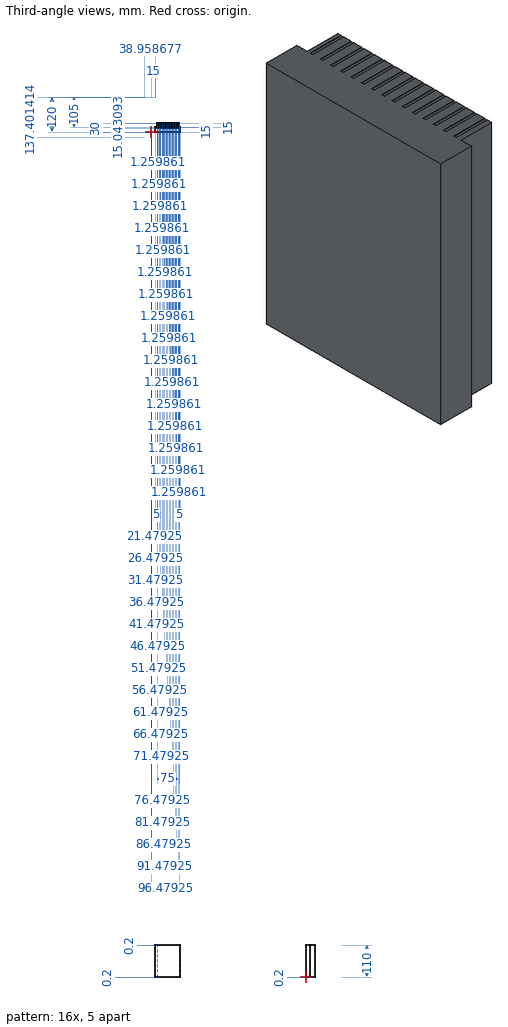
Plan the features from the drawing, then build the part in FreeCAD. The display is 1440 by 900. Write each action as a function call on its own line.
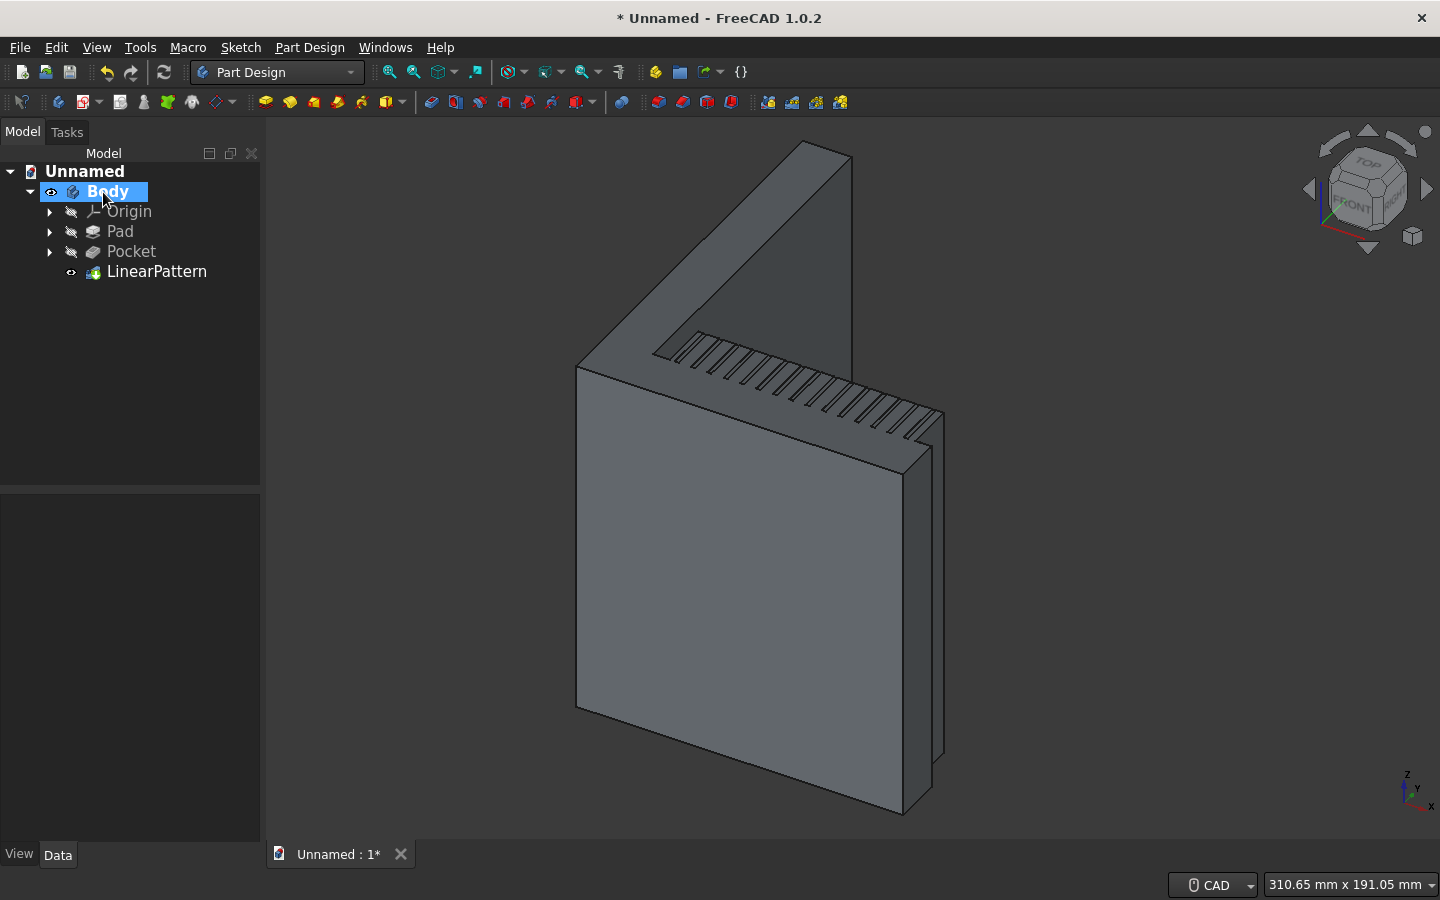
click(50, 212)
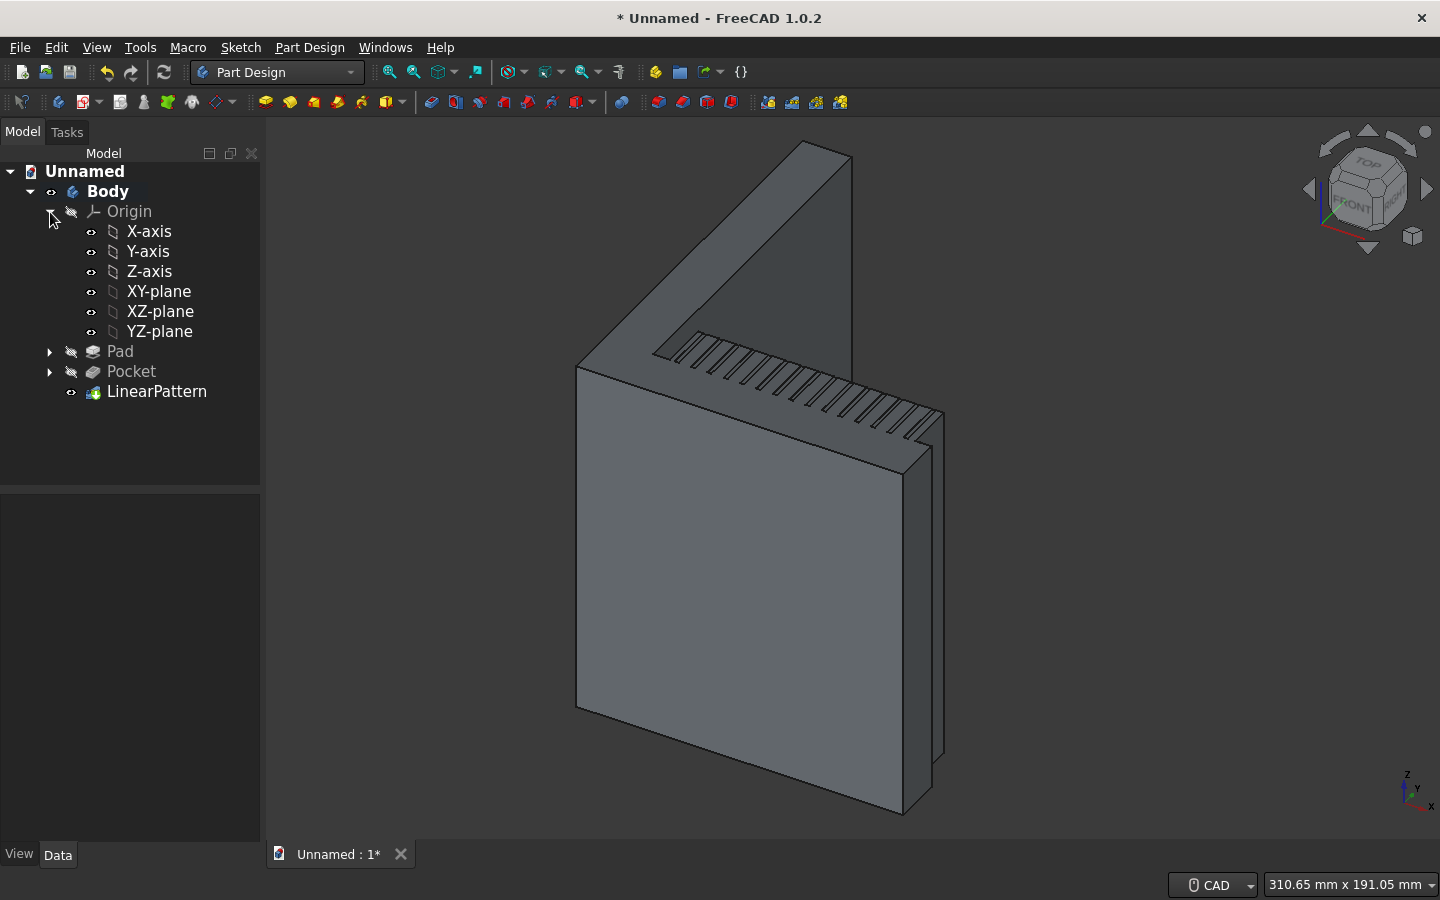
click(136, 292)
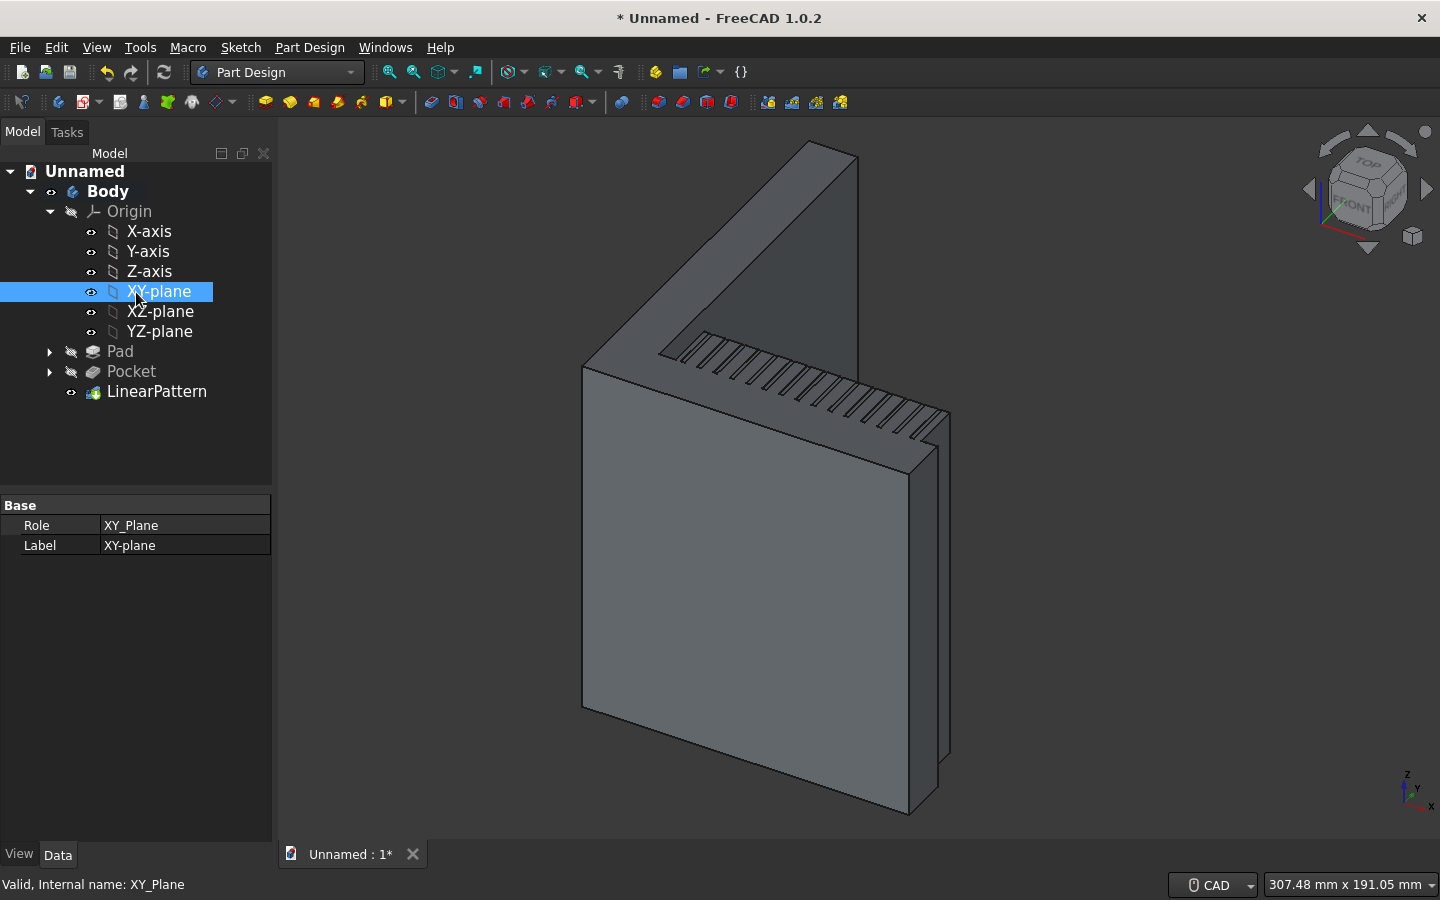
click(216, 102)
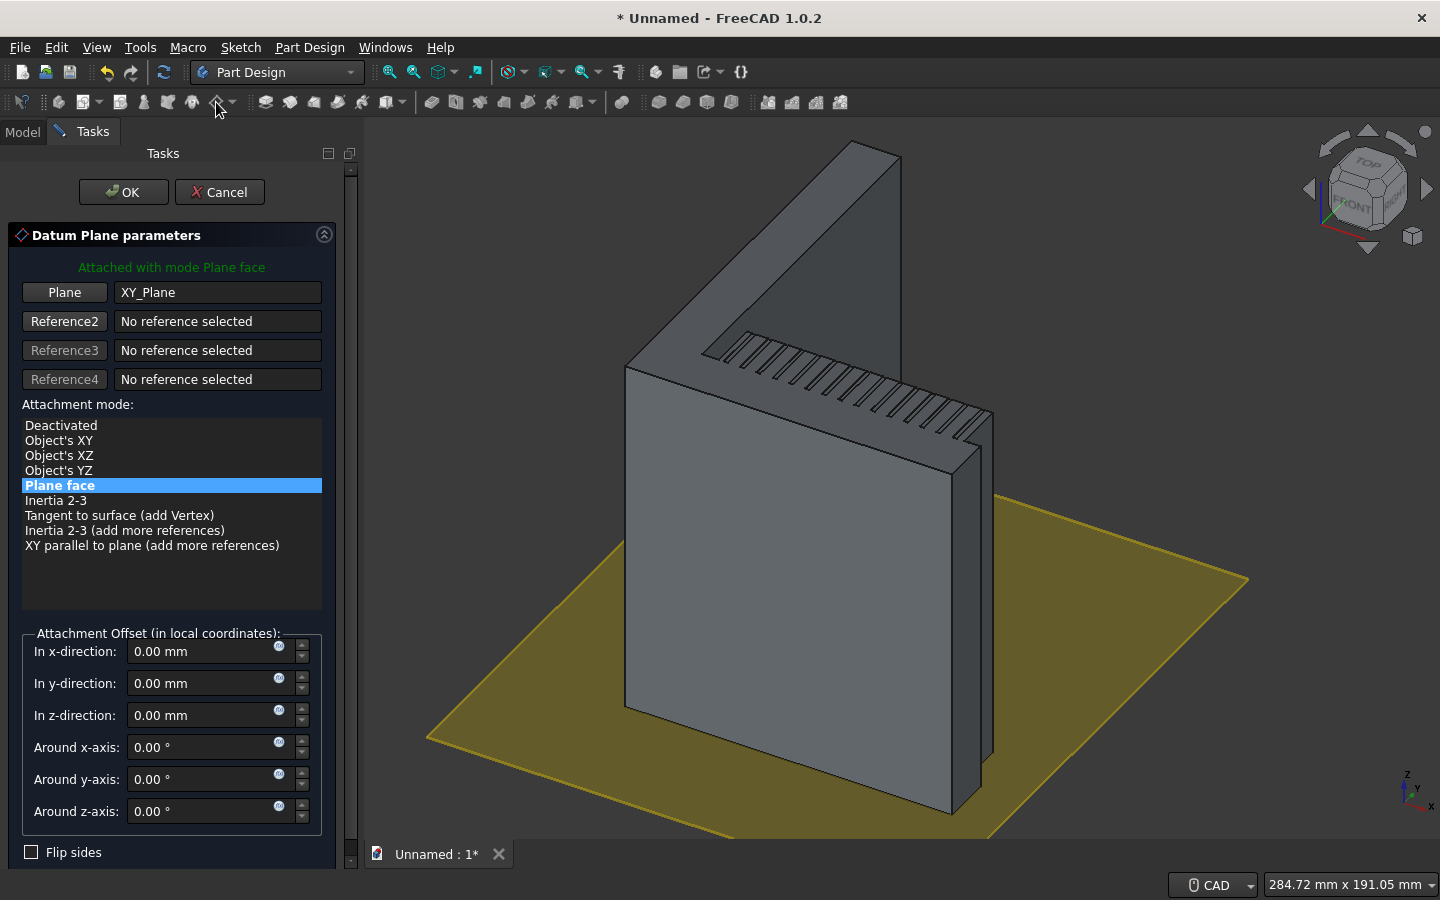
triple_click(210, 715)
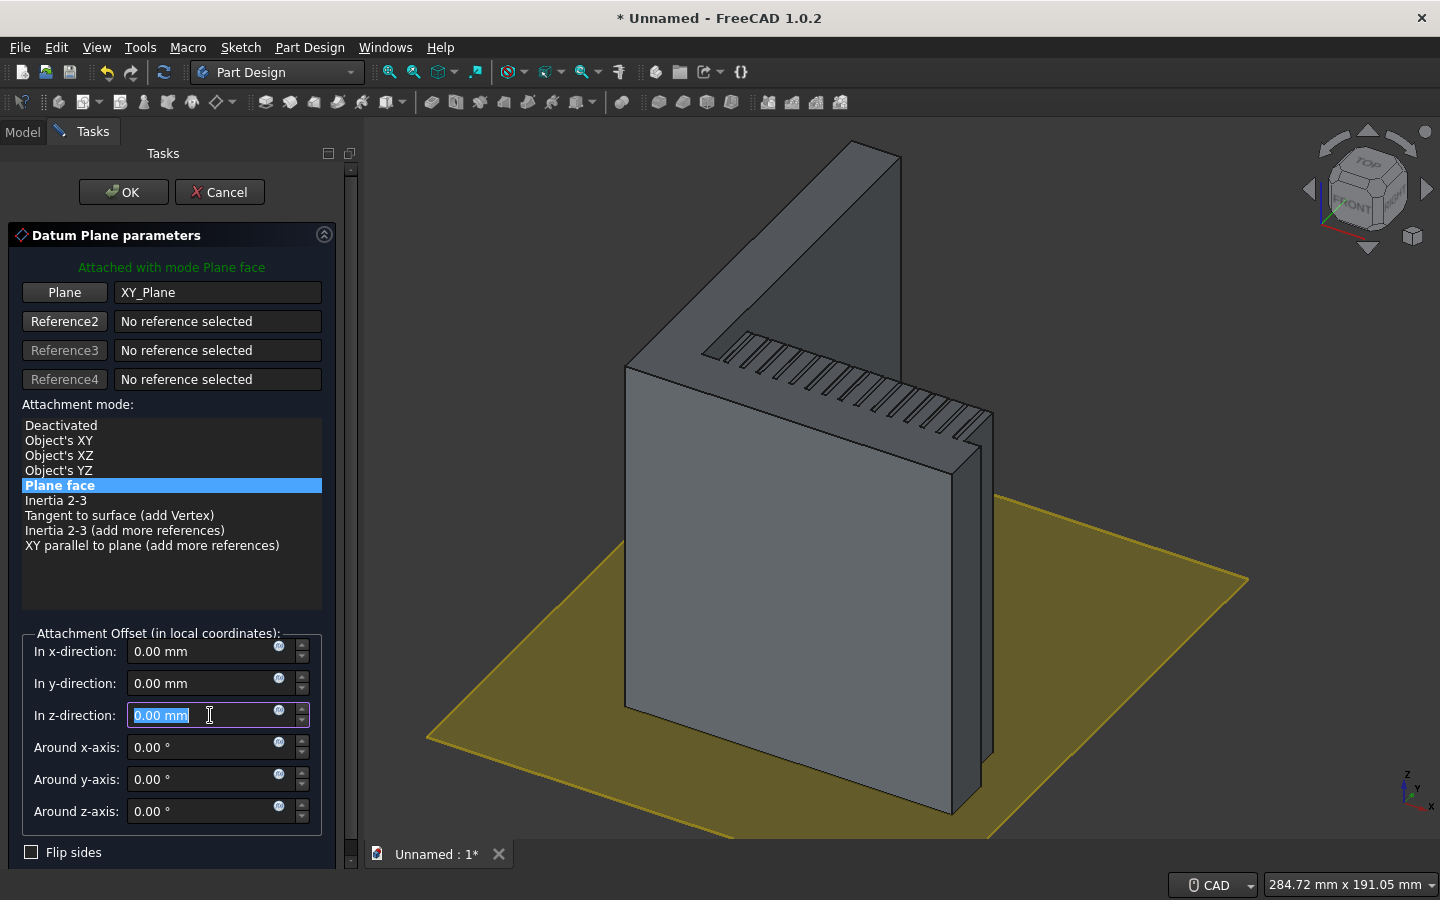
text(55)
key(Tab)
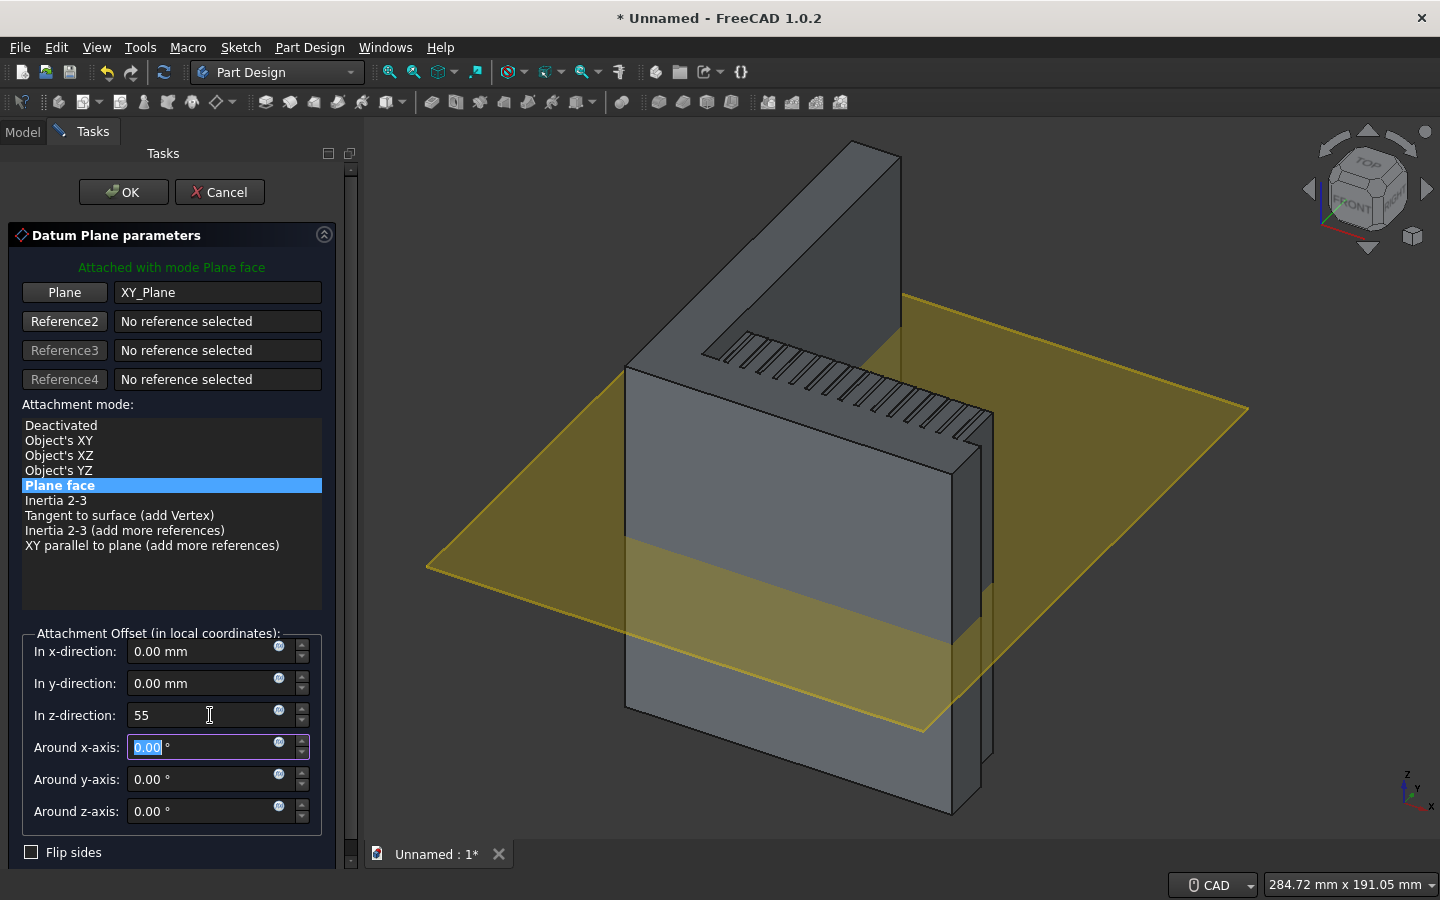
click(124, 192)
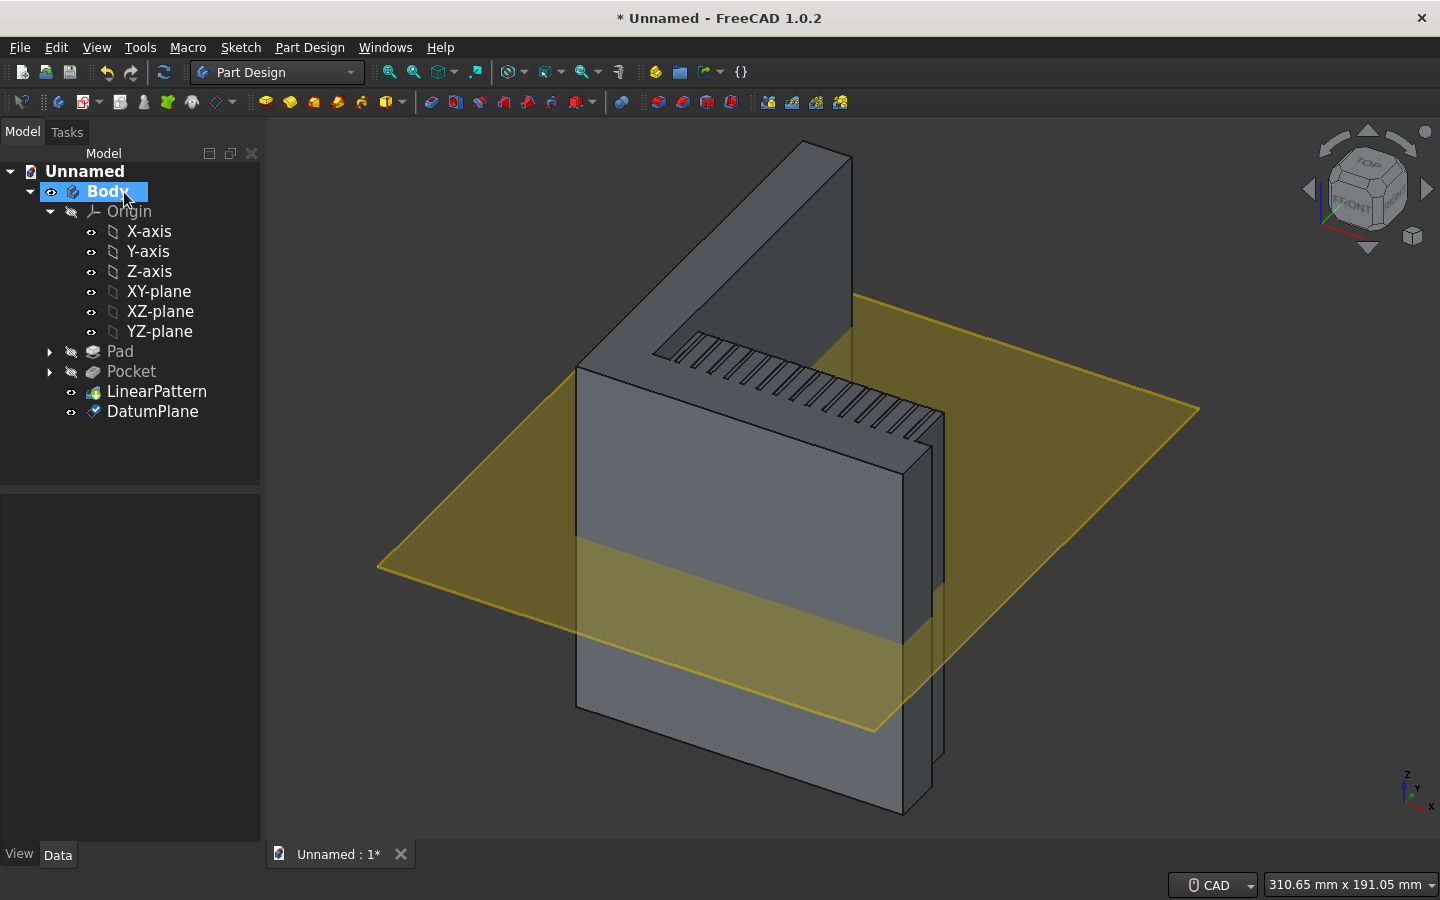
click(116, 372)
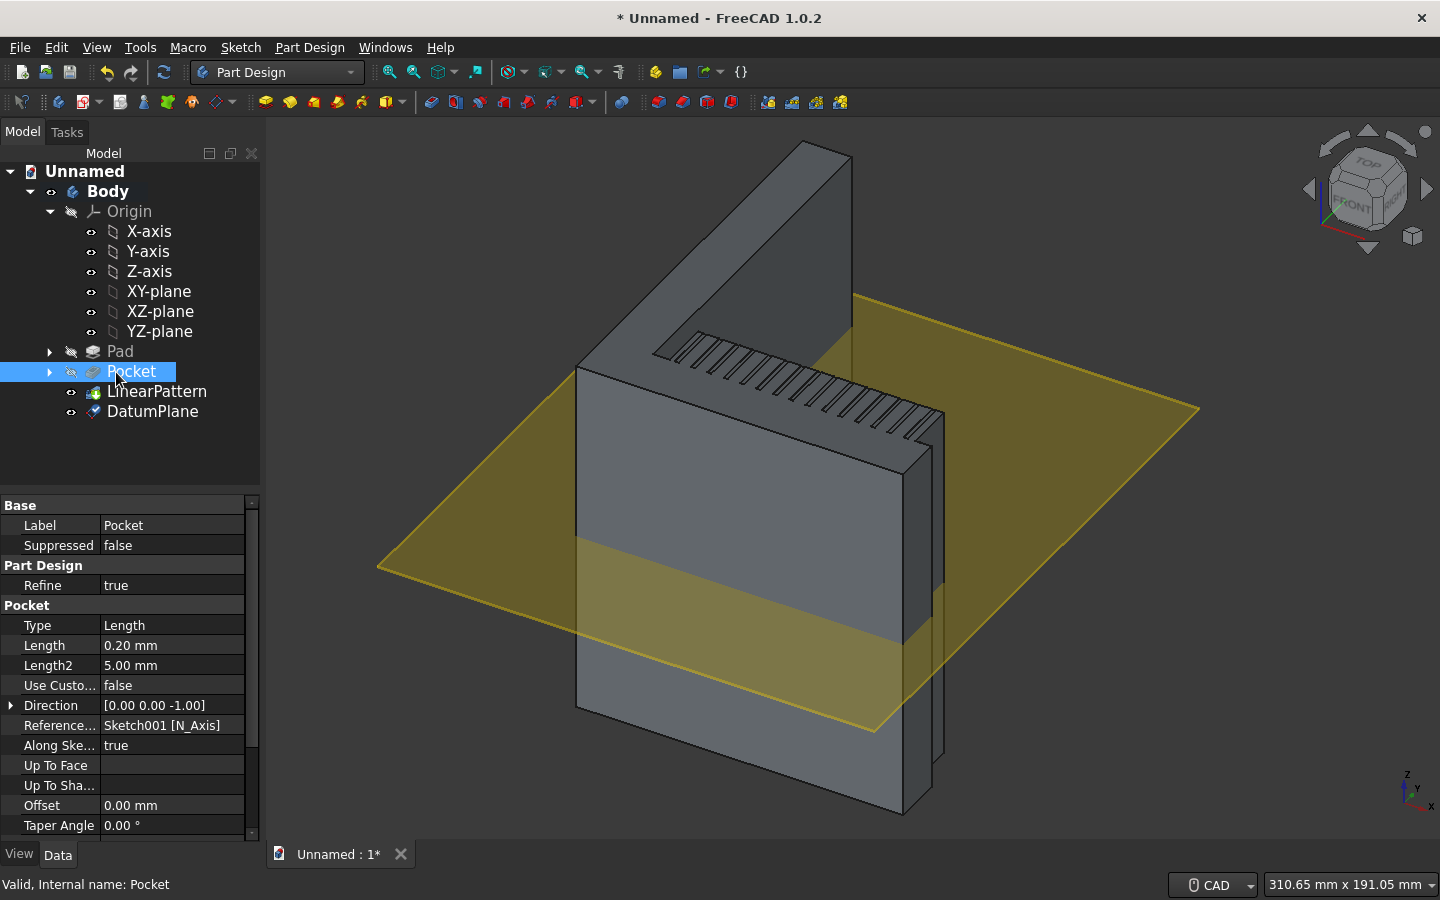
click(768, 102)